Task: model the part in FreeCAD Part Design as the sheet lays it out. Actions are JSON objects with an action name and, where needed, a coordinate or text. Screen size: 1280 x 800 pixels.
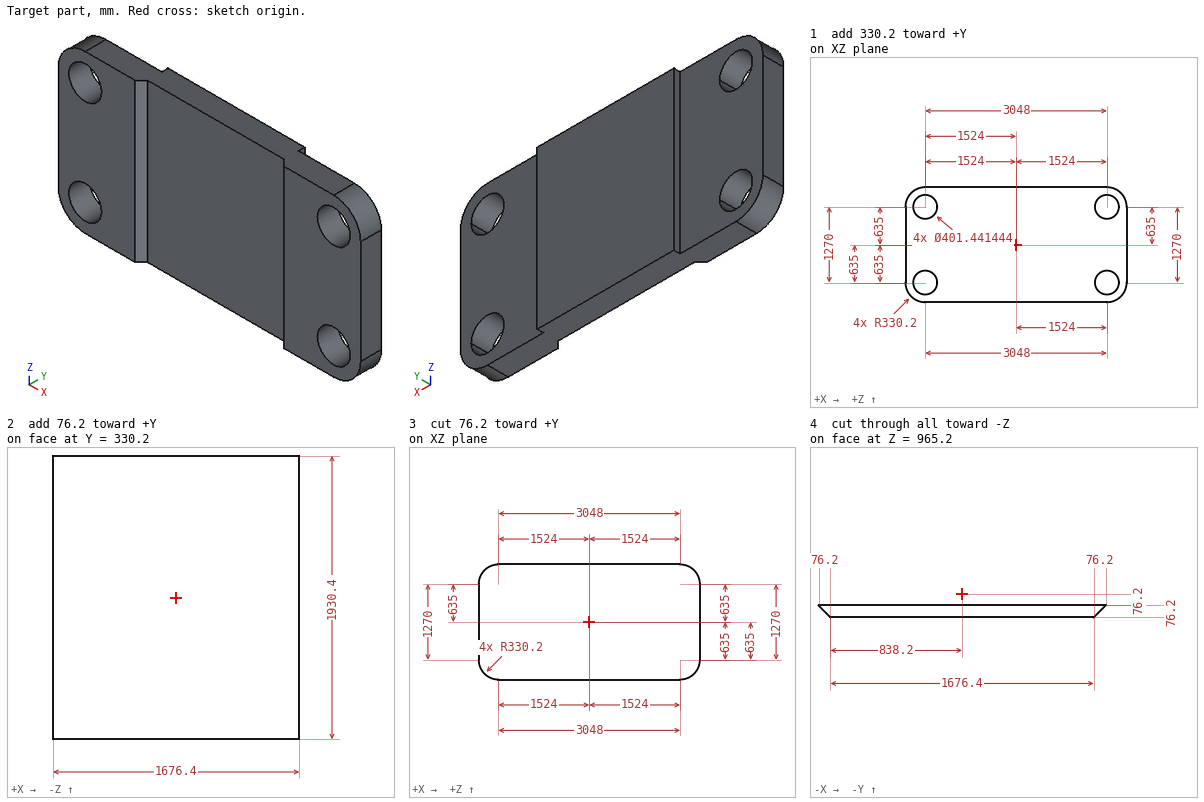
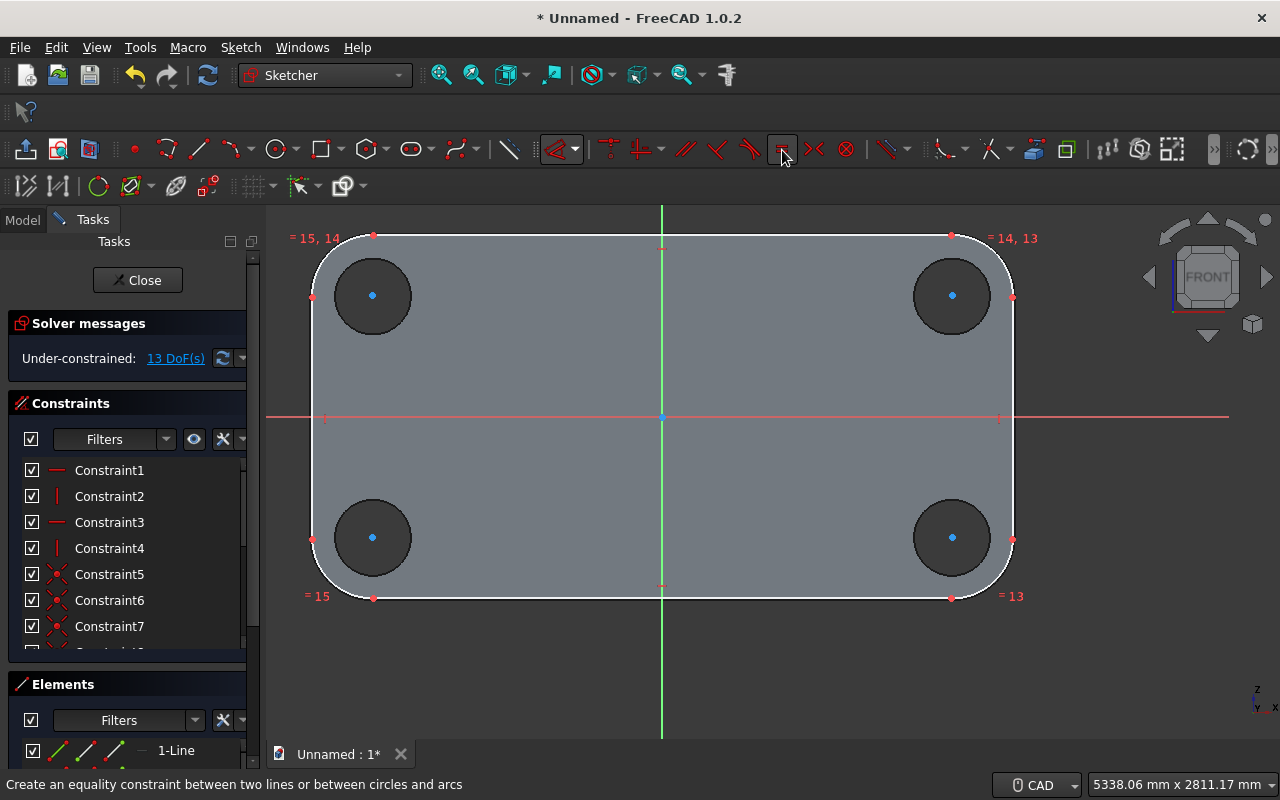
{"action": "left_click", "coordinate": [979, 592]}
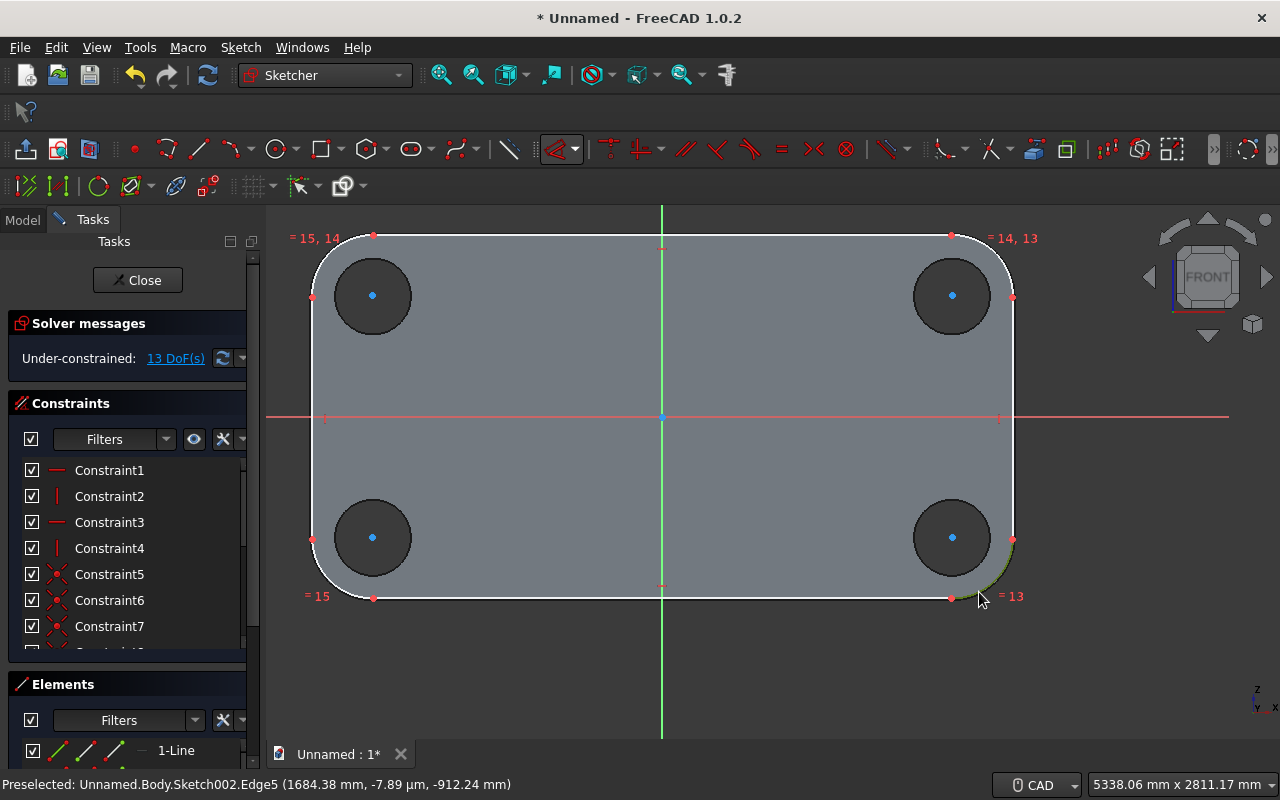
{"action": "key", "text": "k r"}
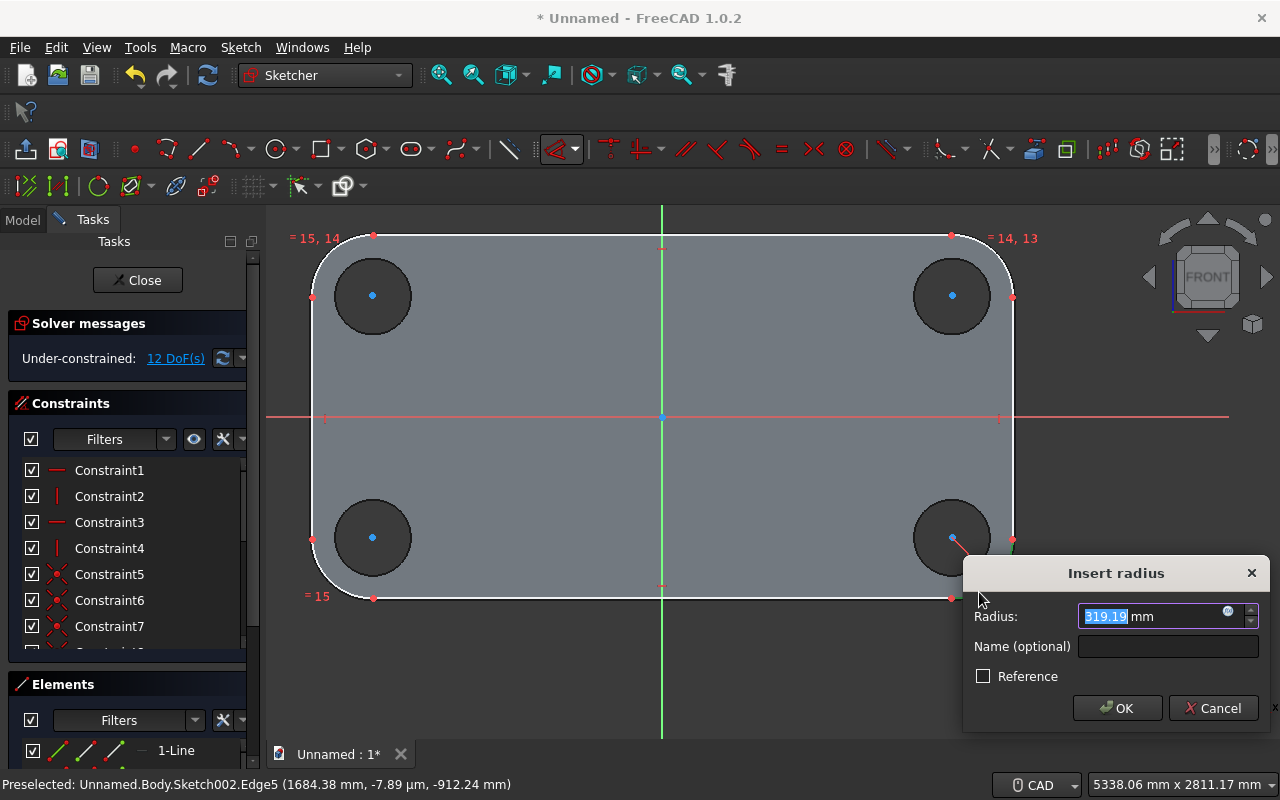
{"action": "type", "text": "330.2"}
{"action": "key", "text": "Return"}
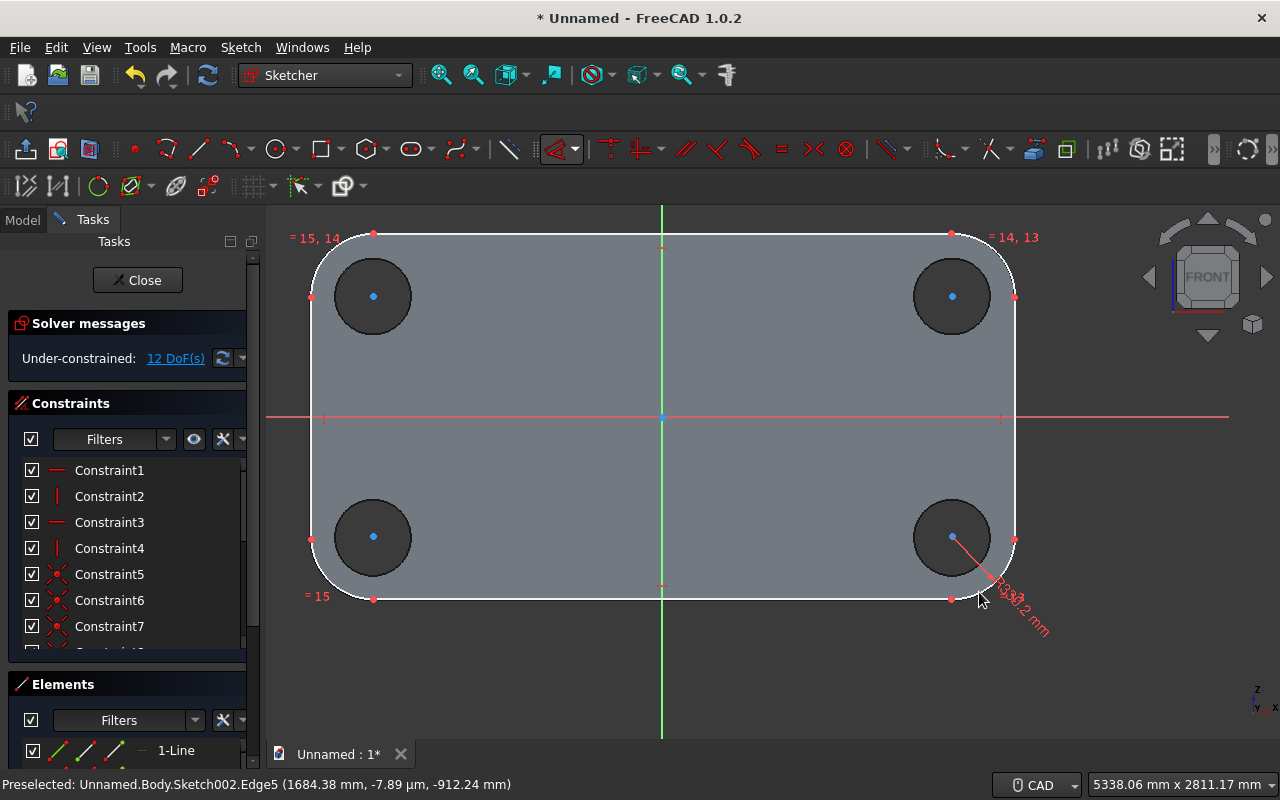
{"action": "left_click", "coordinate": [547, 599]}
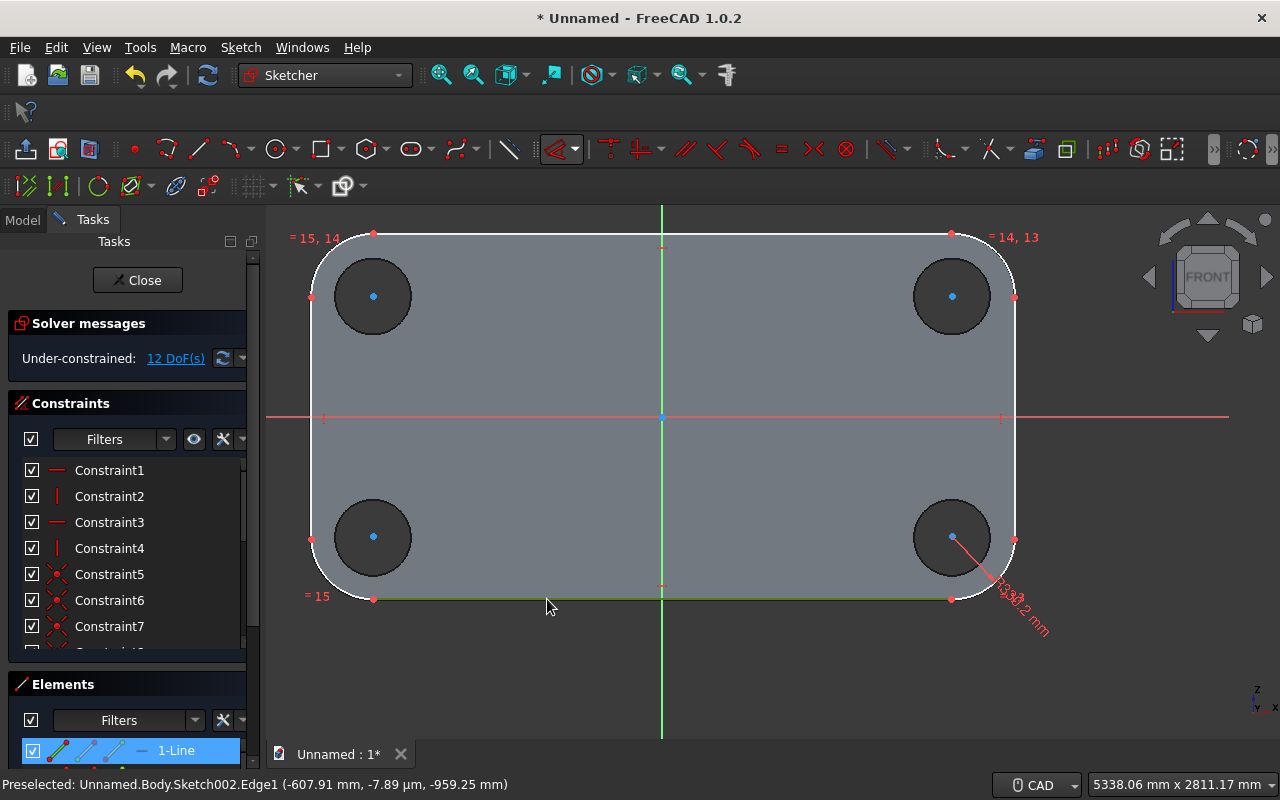
{"action": "key", "text": "l"}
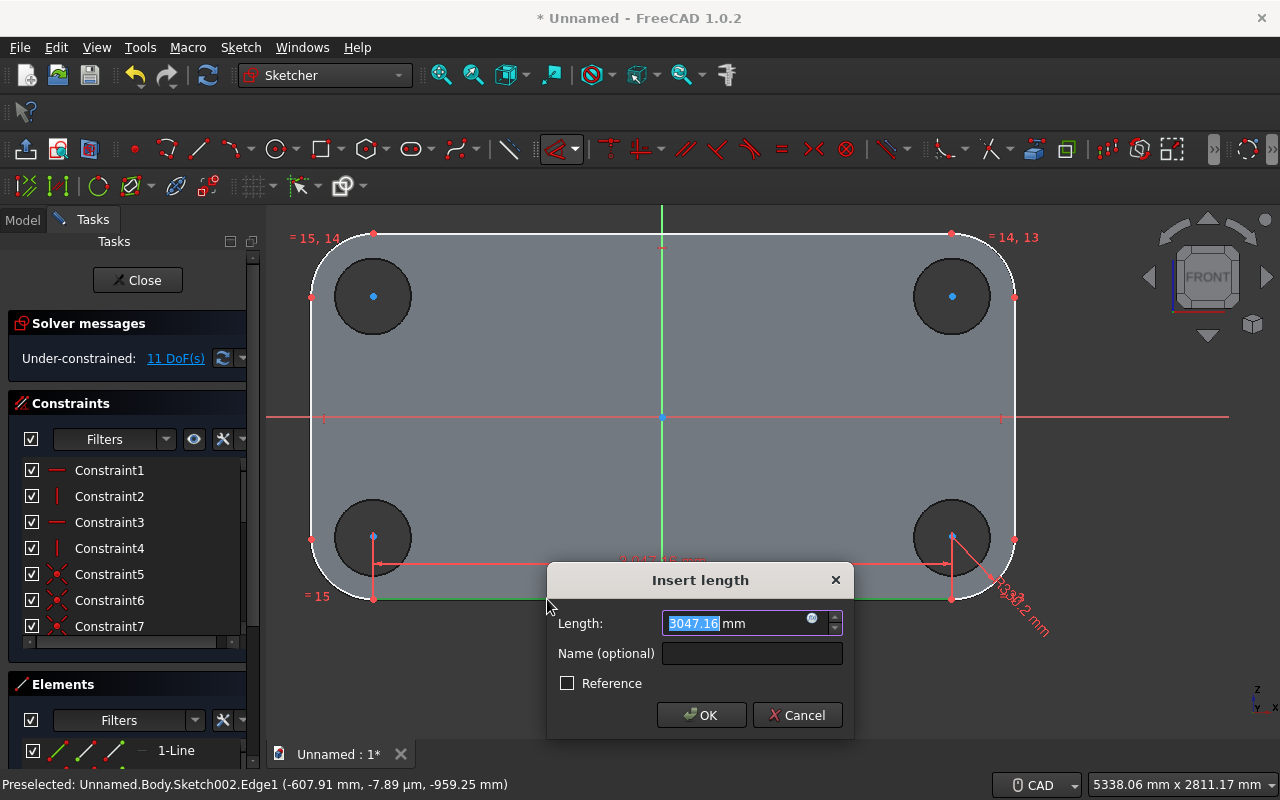
{"action": "type", "text": "3048"}
{"action": "key", "text": "Return"}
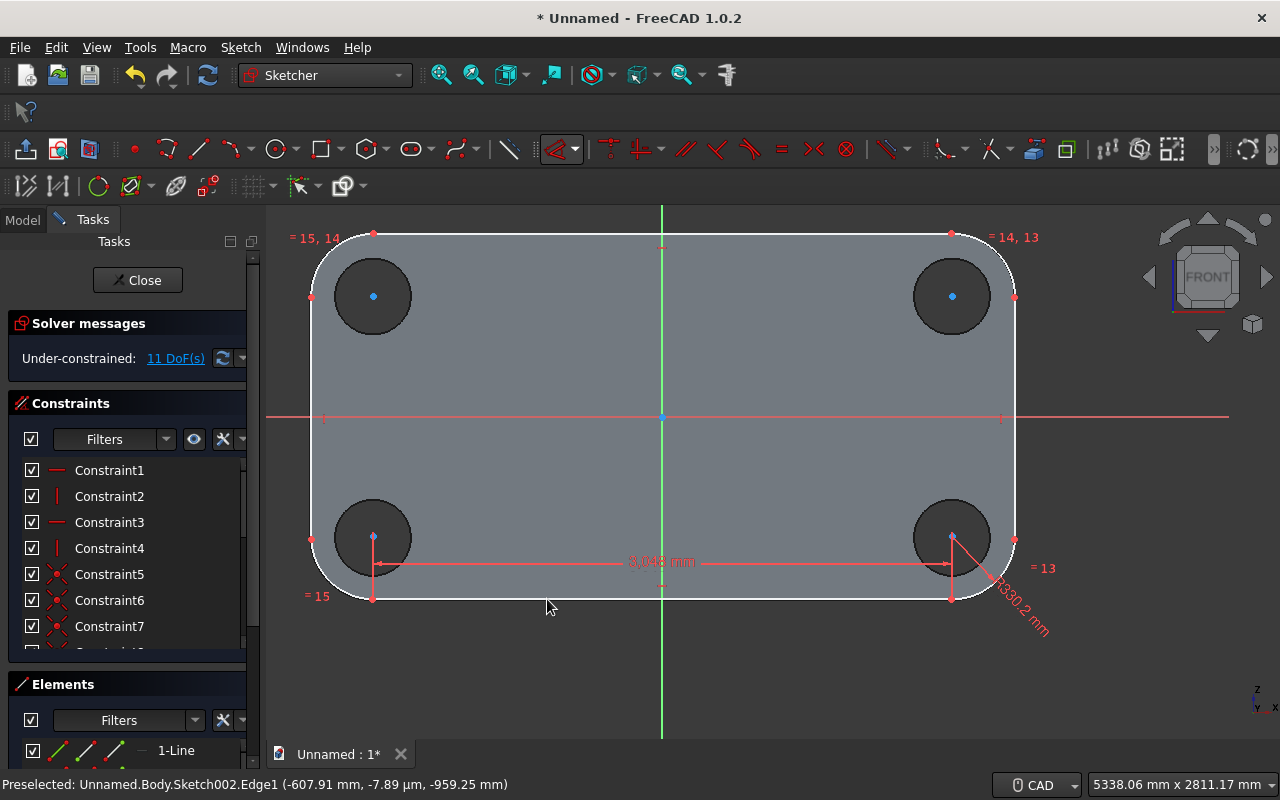
{"action": "left_click", "coordinate": [1015, 467]}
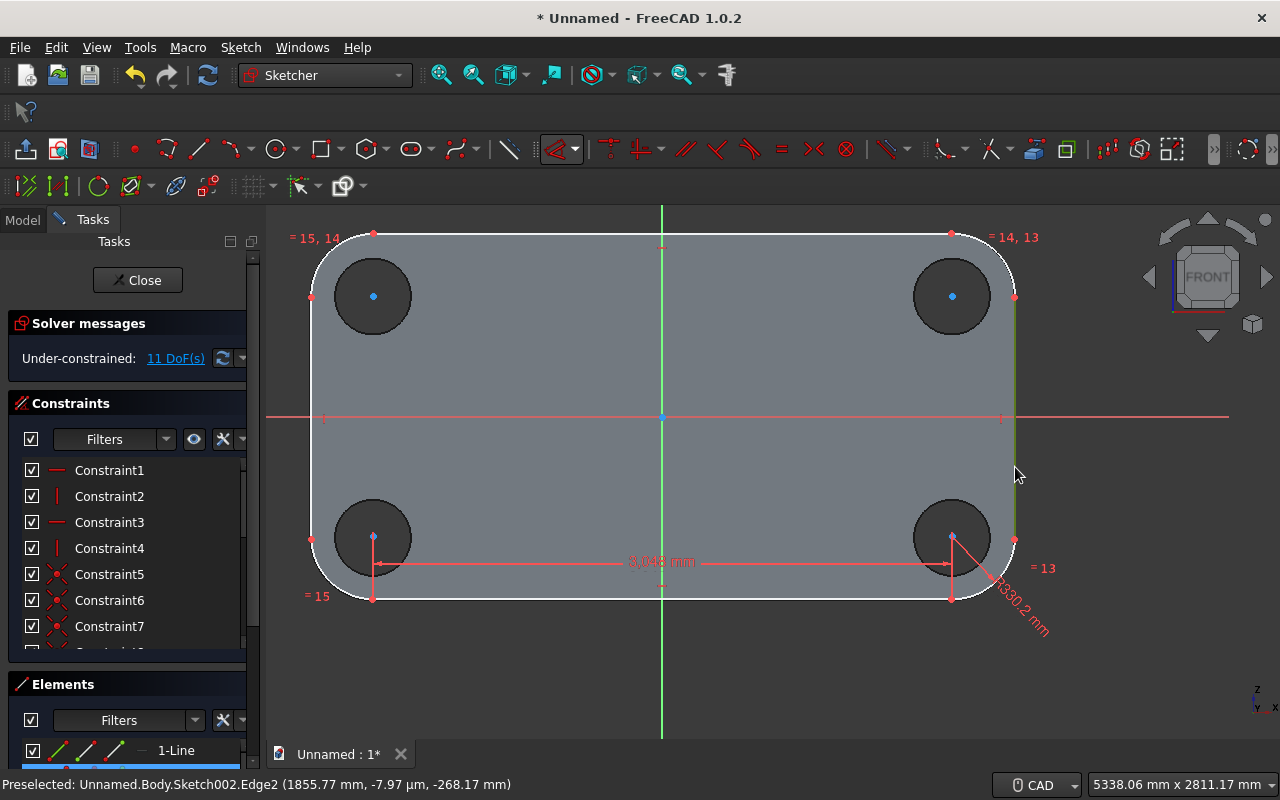
{"action": "key", "text": "i"}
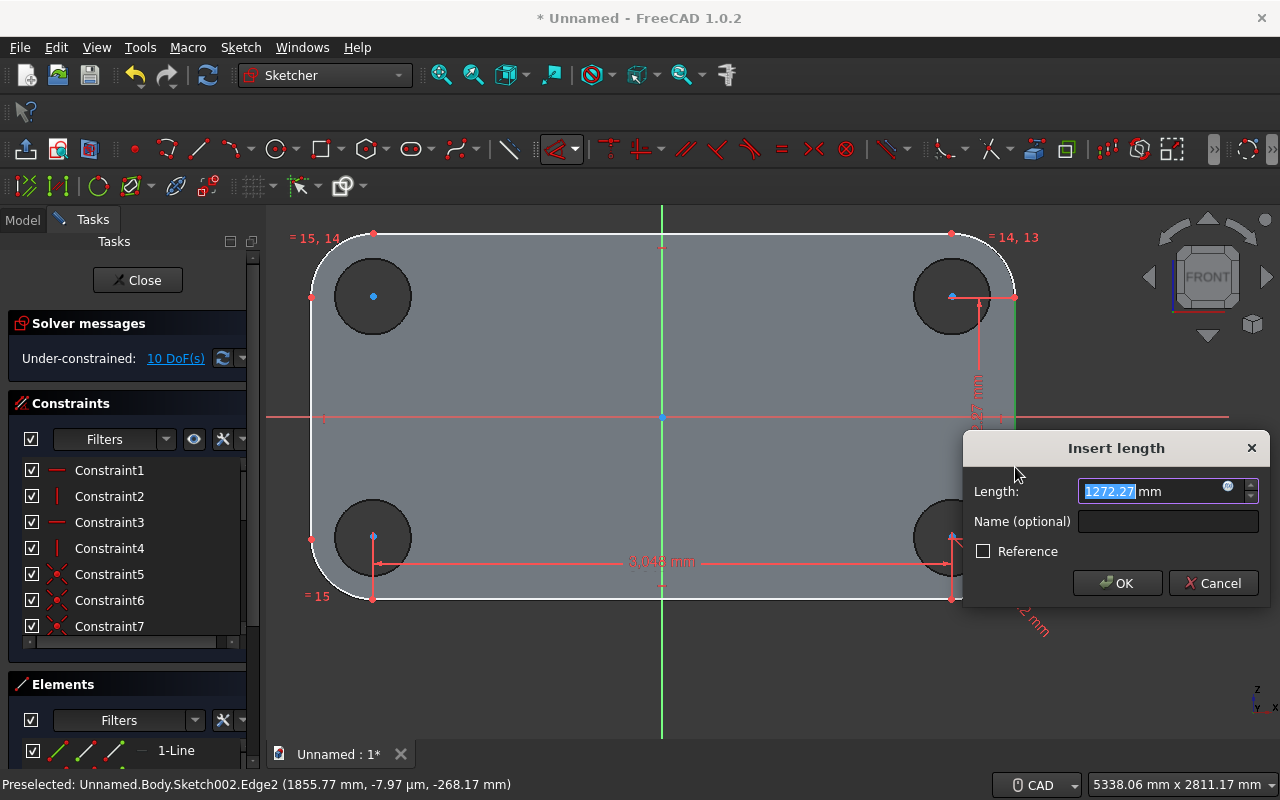
{"action": "type", "text": "1270"}
{"action": "key", "text": "Return"}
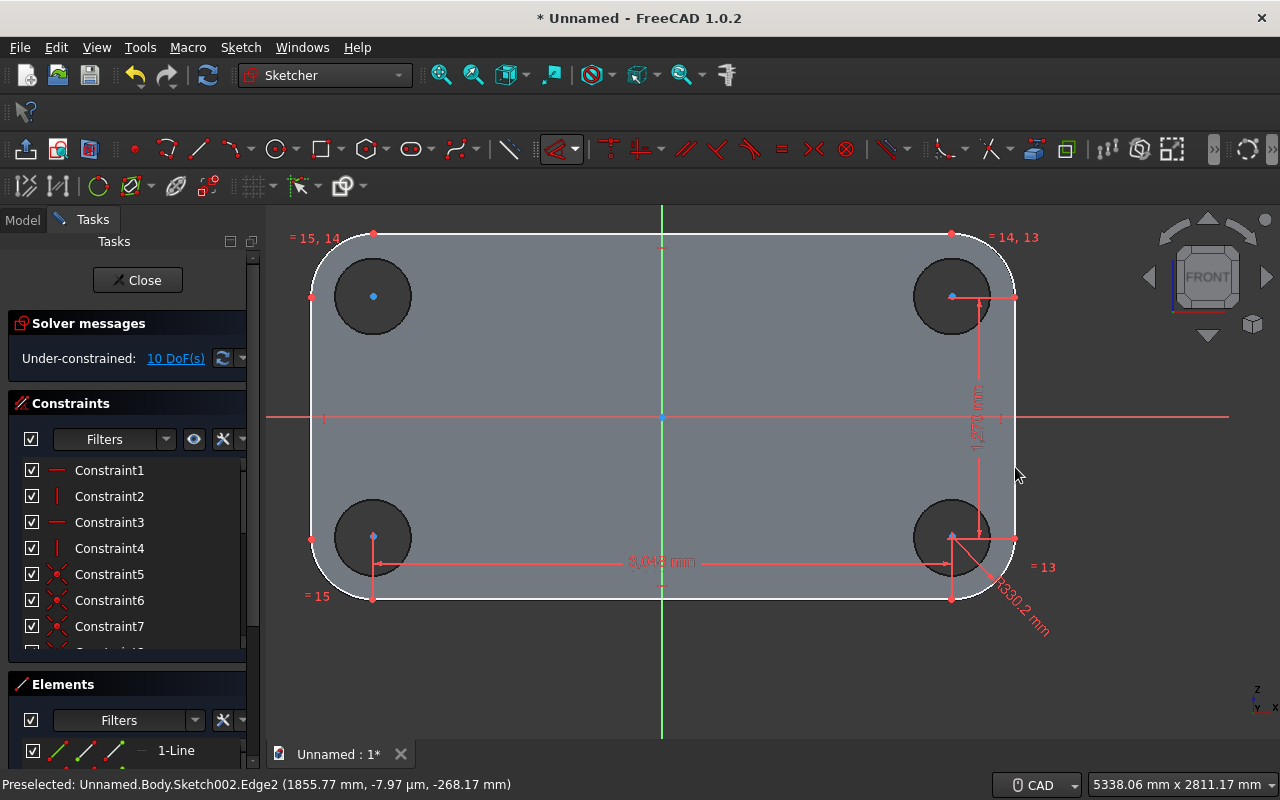
{"action": "left_click", "coordinate": [778, 234]}